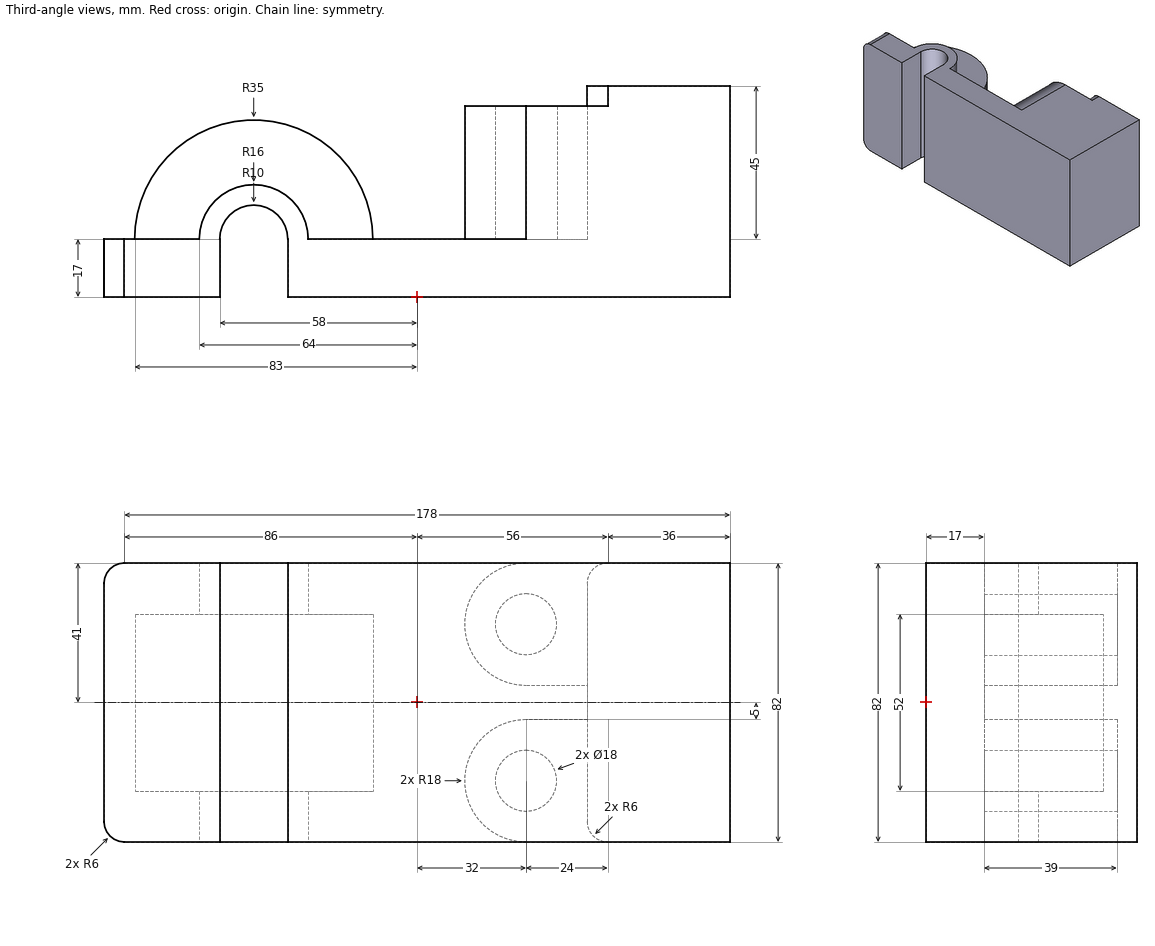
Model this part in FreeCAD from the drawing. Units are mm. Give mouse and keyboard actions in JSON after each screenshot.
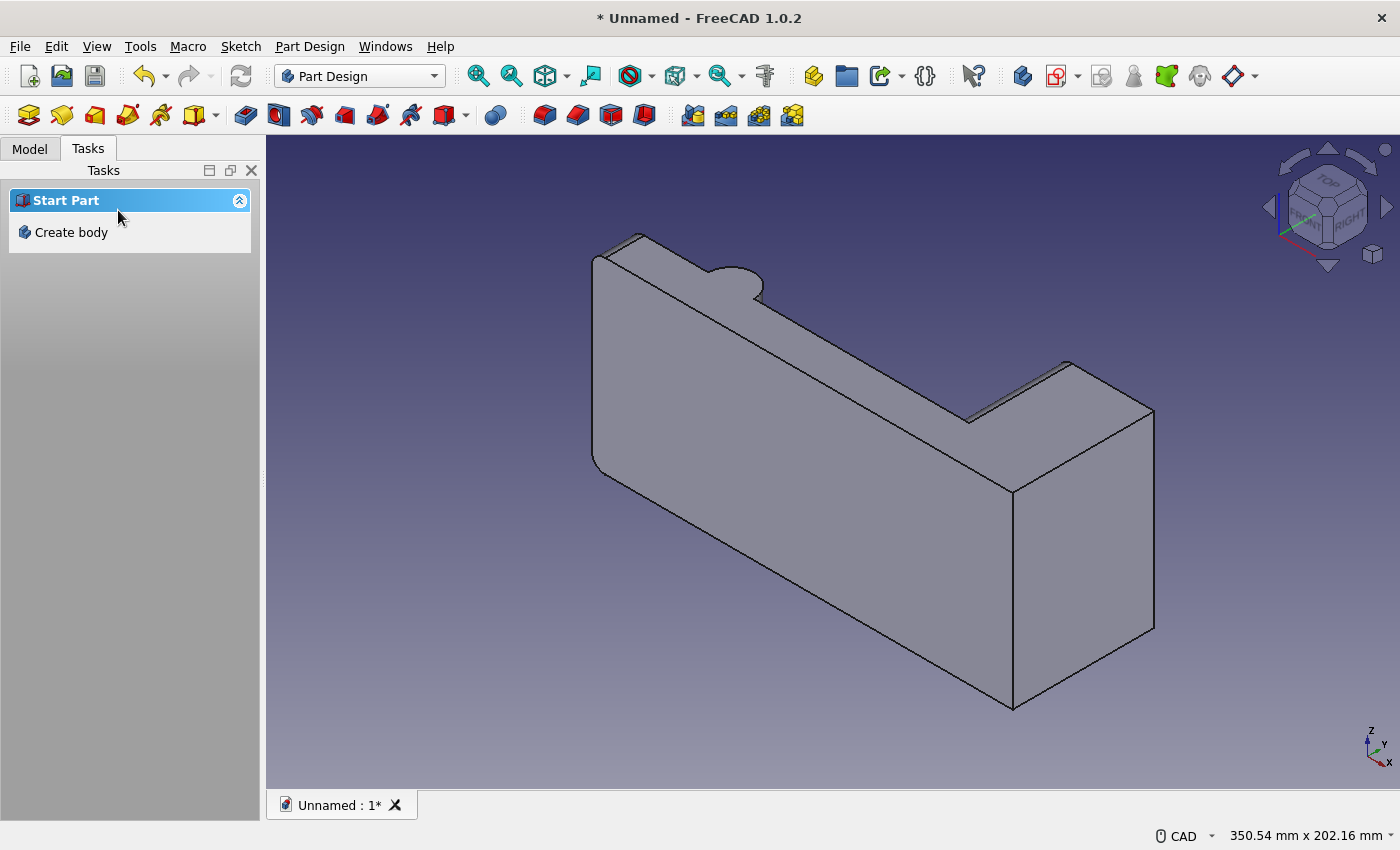
{"action": "left_click", "coordinate": [1095, 411]}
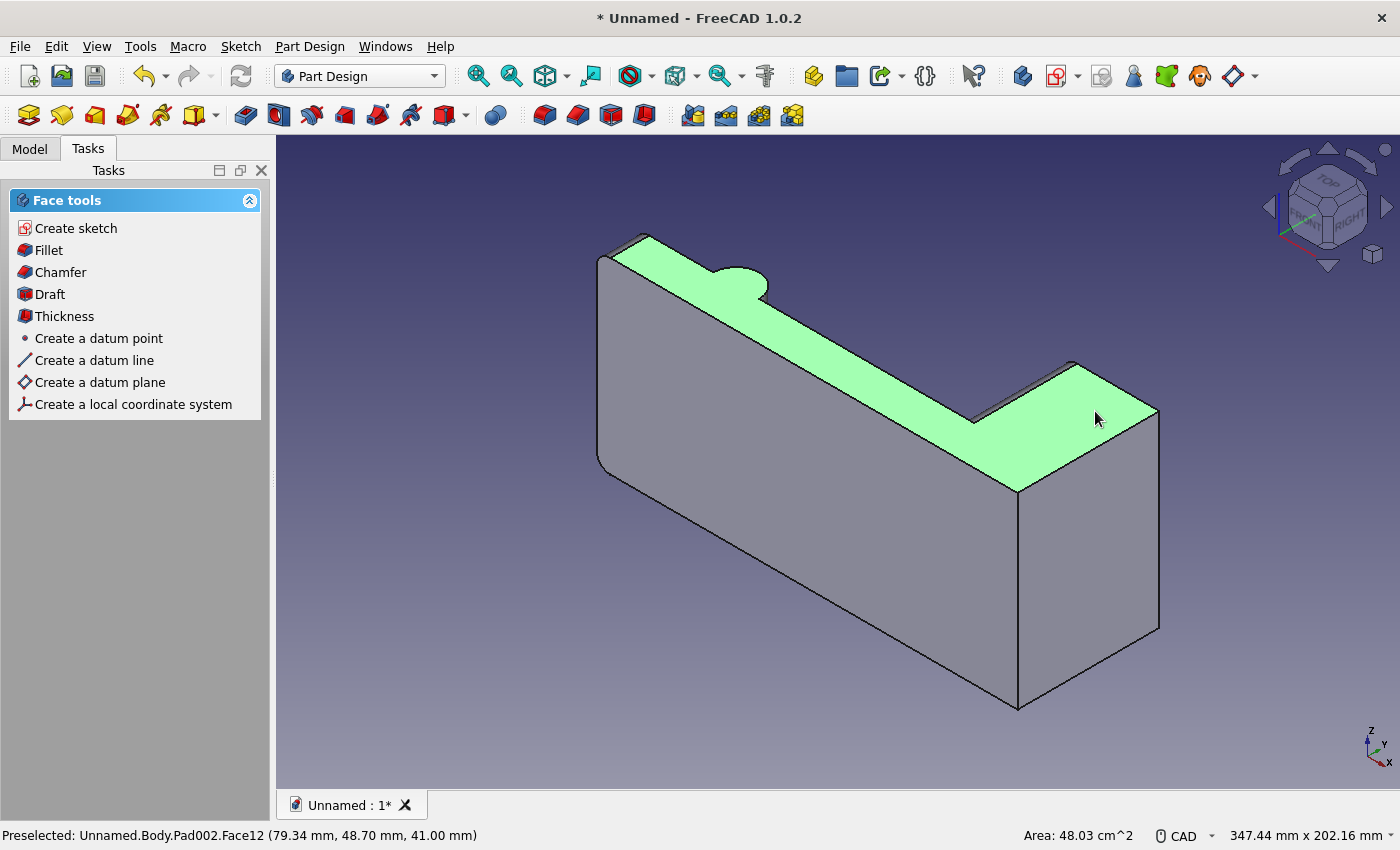
{"action": "left_click", "coordinate": [1056, 76]}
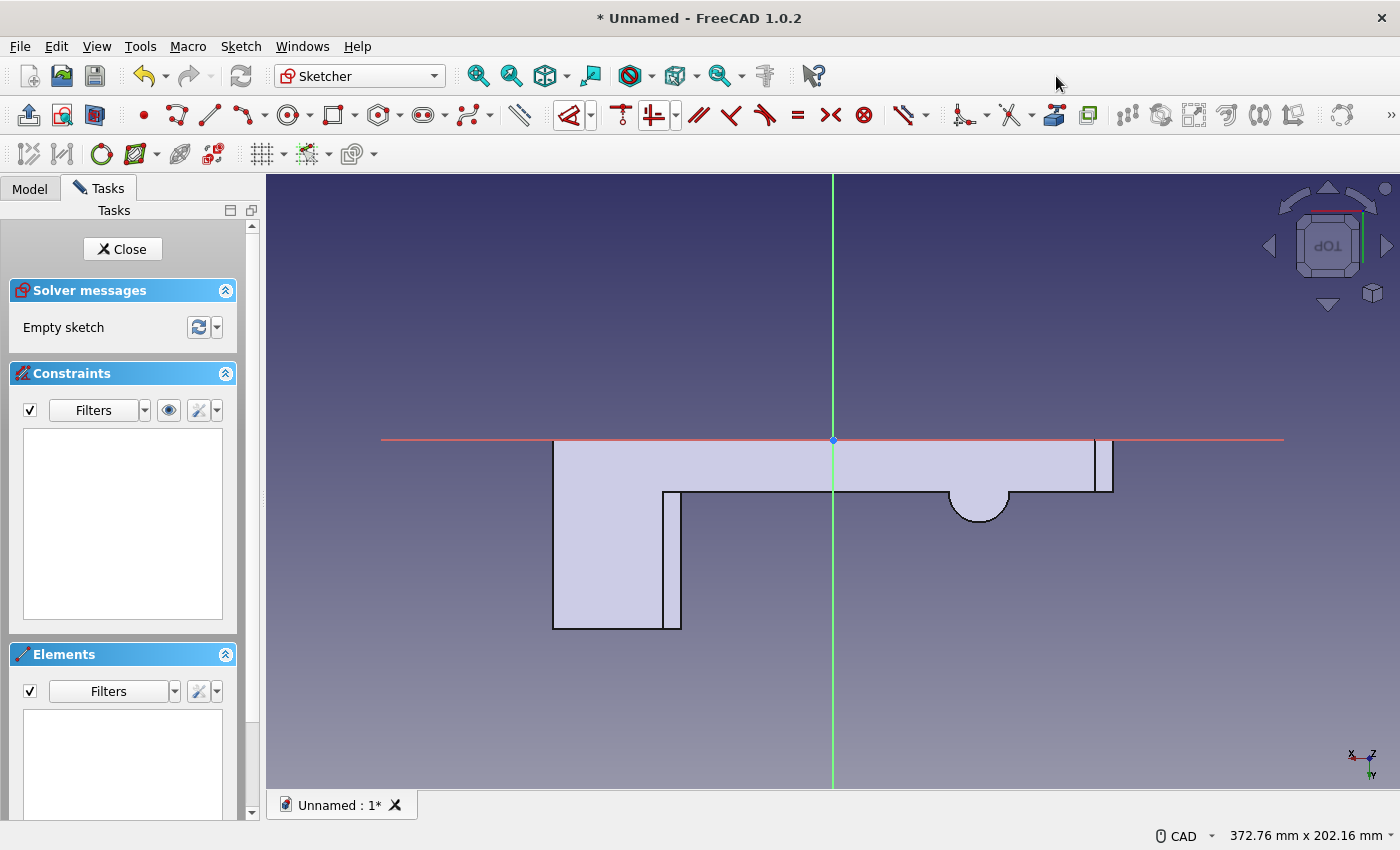
{"action": "scroll", "coordinate": [1002, 495], "scroll_direction": "up", "scroll_amount": 6}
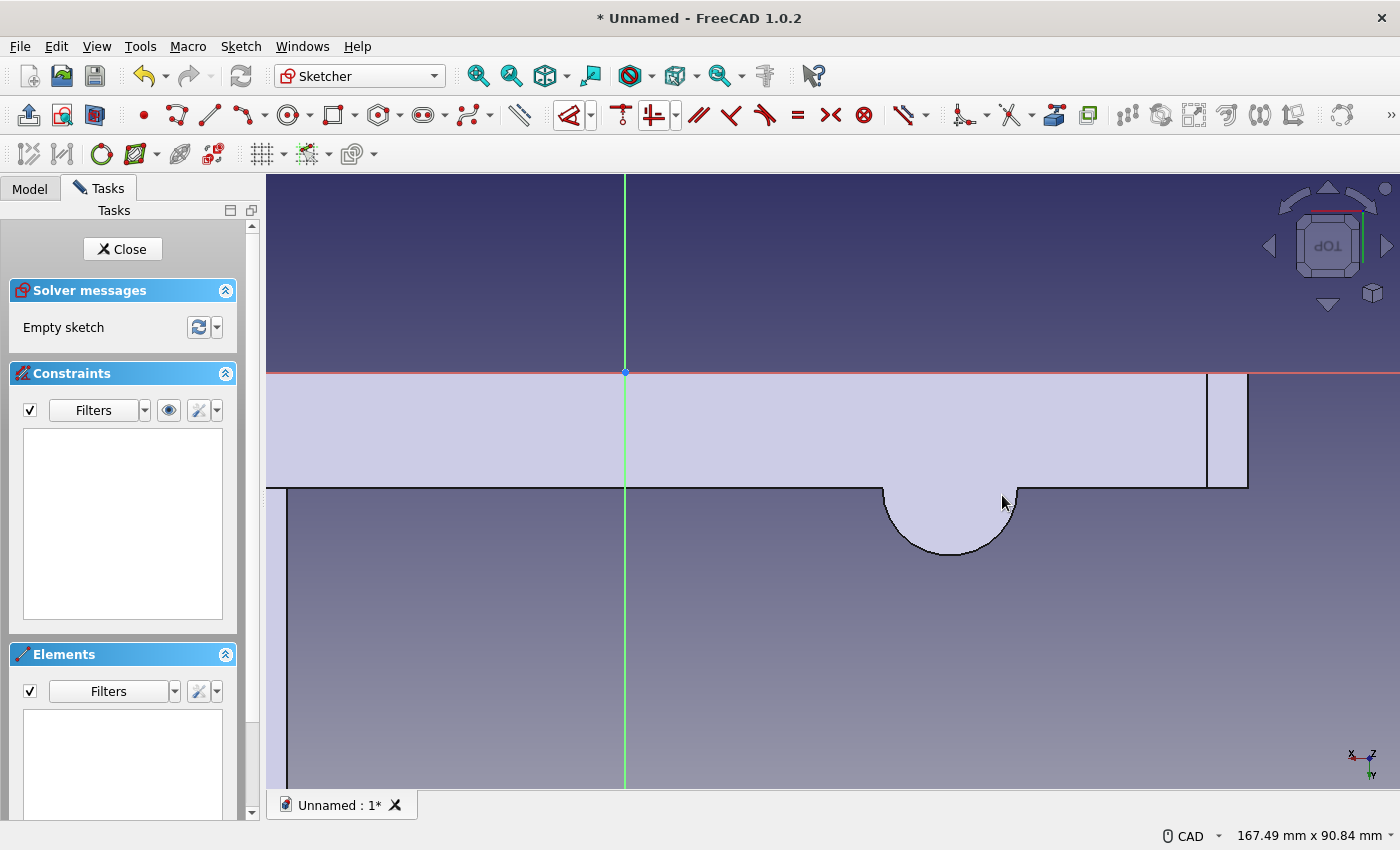
{"action": "left_click", "coordinate": [210, 116]}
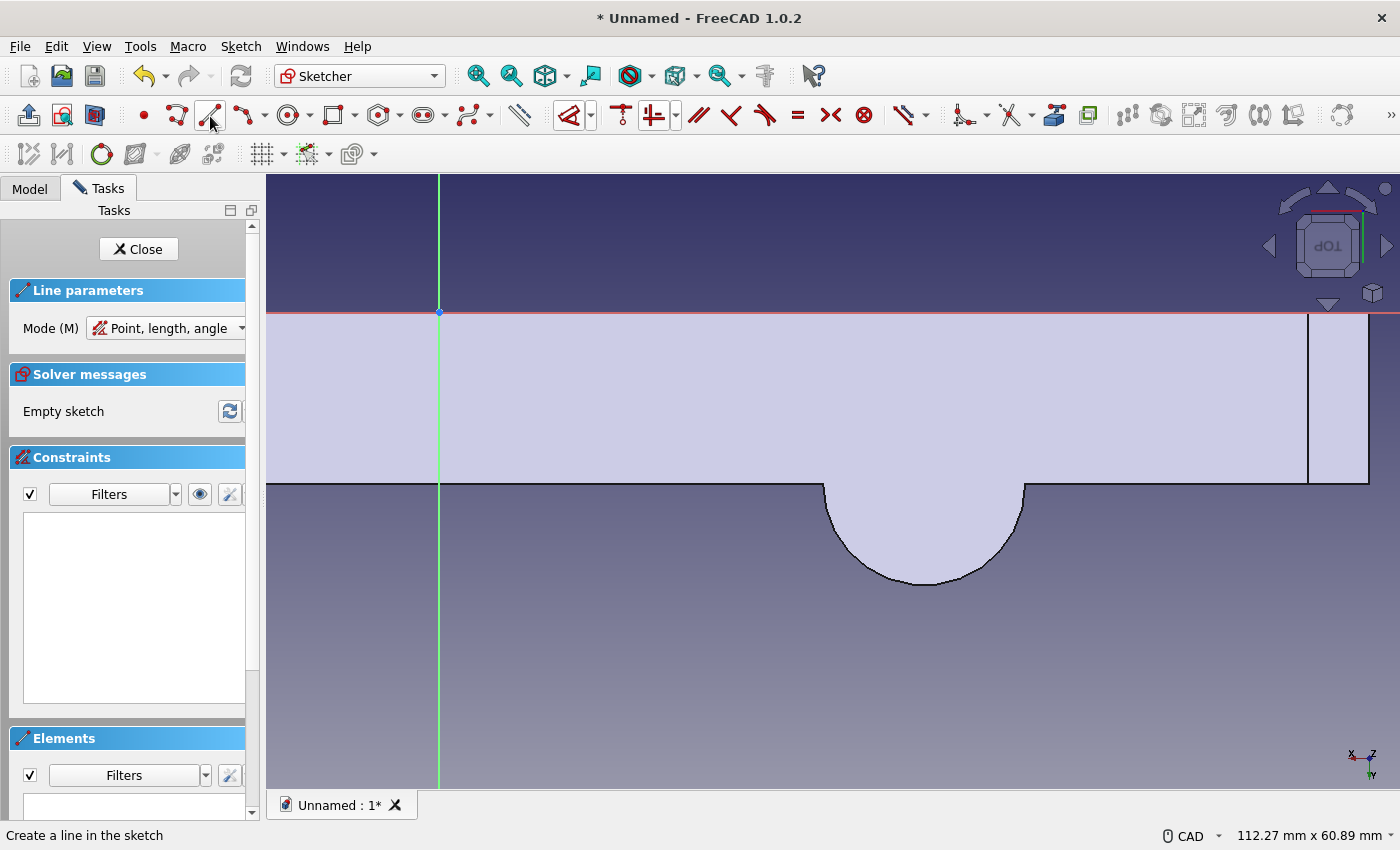
{"action": "left_click", "coordinate": [1086, 484]}
{"action": "left_click", "coordinate": [1025, 484]}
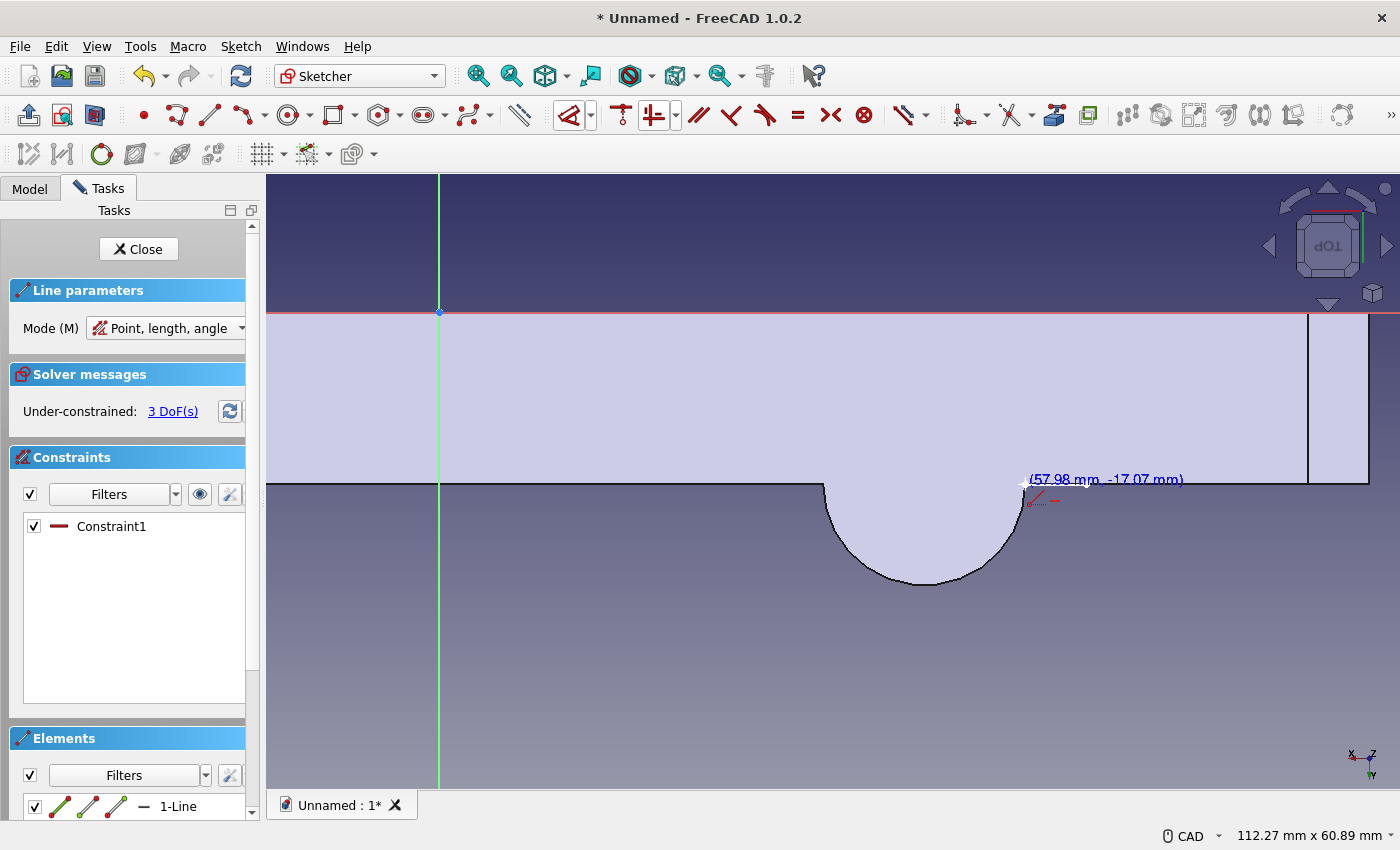
{"action": "left_click", "coordinate": [823, 484]}
{"action": "left_click", "coordinate": [763, 484]}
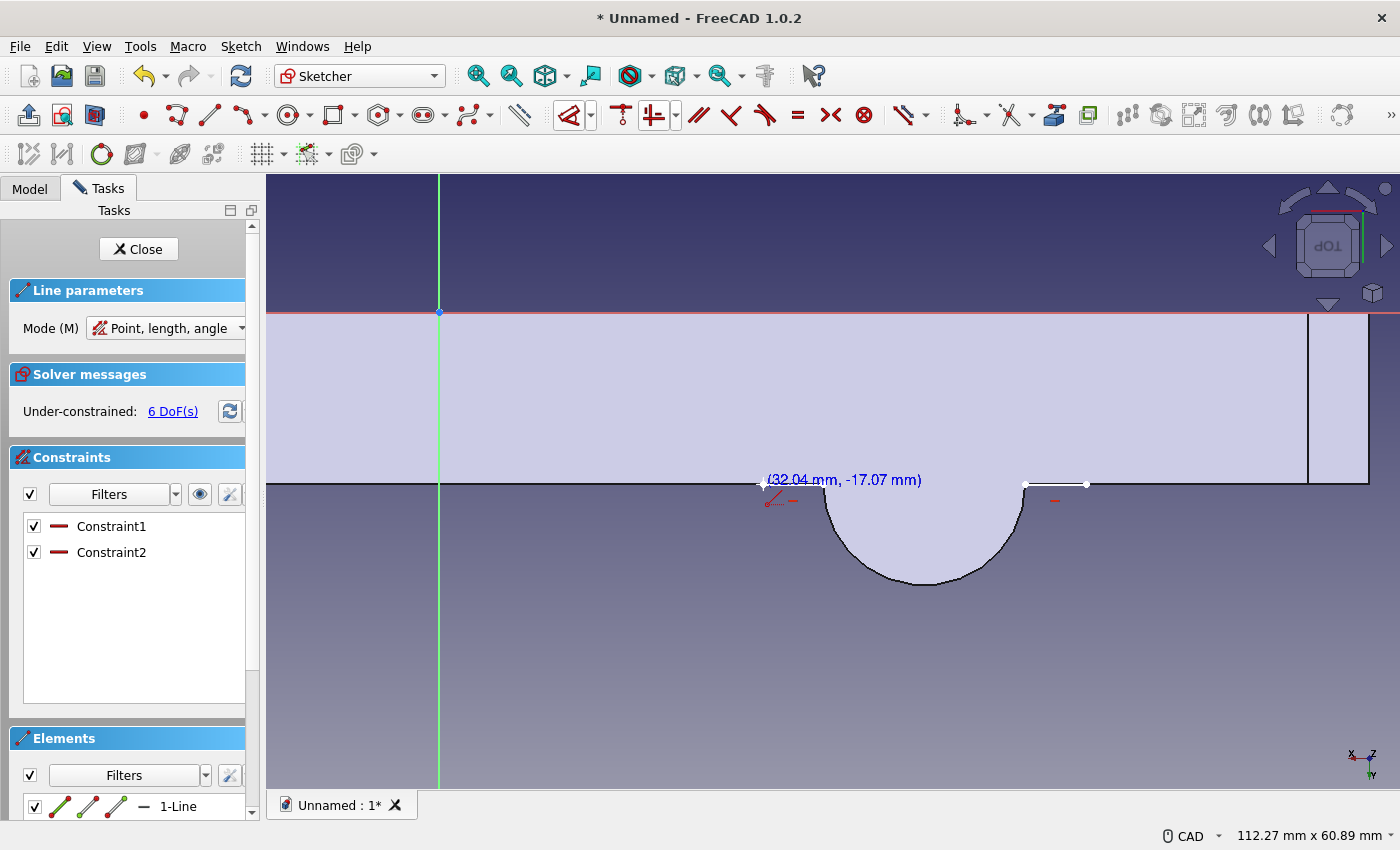
{"action": "left_click", "coordinate": [242, 116]}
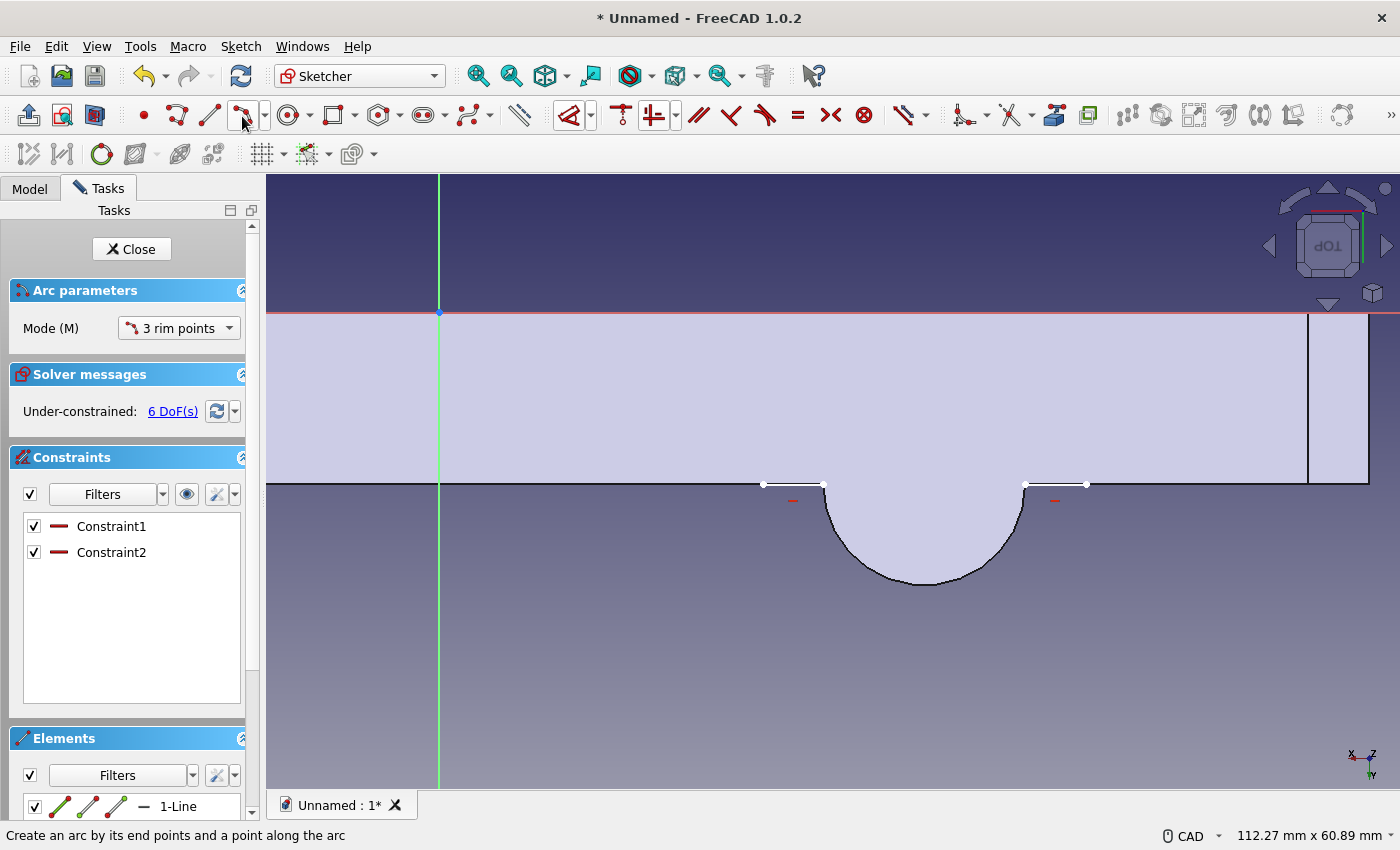
{"action": "left_click", "coordinate": [1025, 485]}
{"action": "left_click", "coordinate": [823, 485]}
{"action": "left_click", "coordinate": [924, 585]}